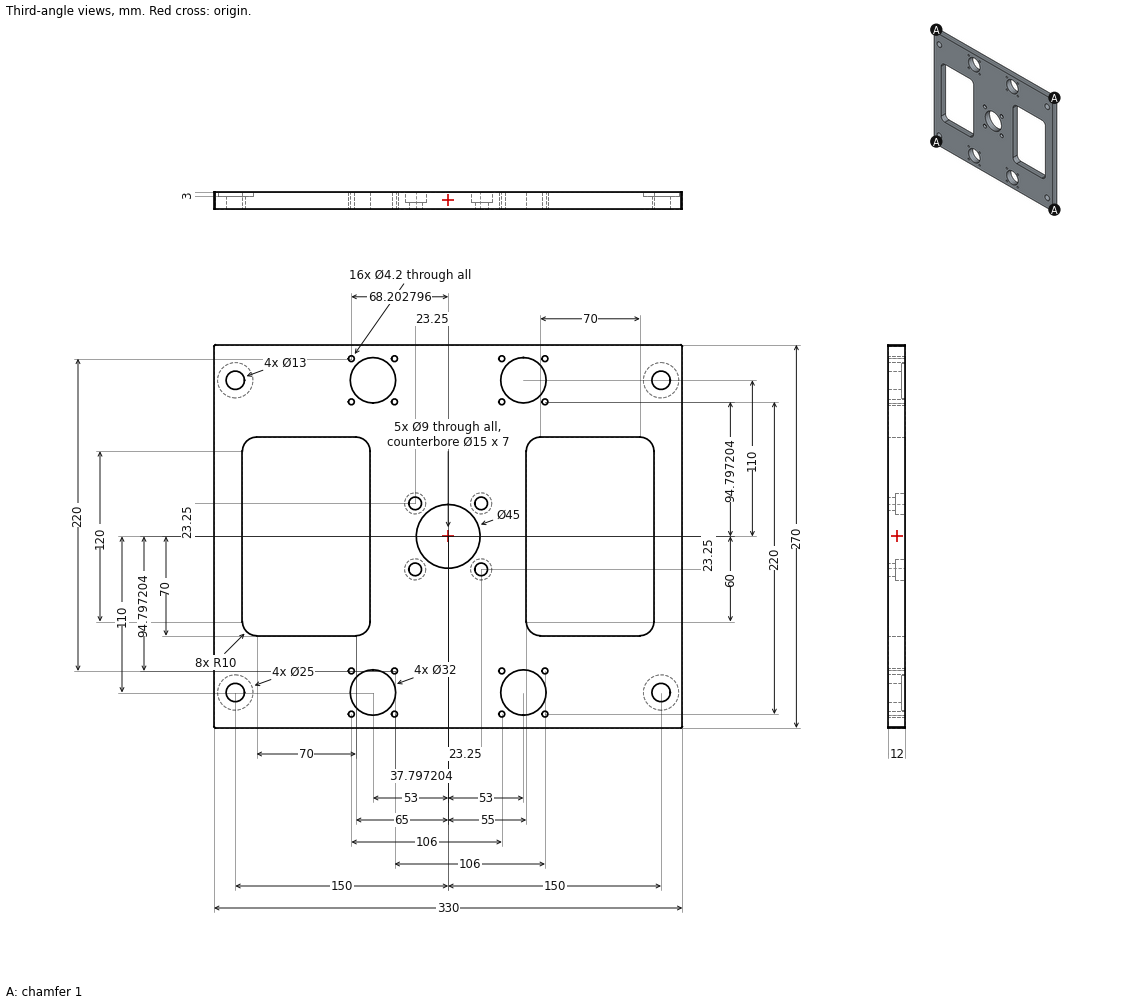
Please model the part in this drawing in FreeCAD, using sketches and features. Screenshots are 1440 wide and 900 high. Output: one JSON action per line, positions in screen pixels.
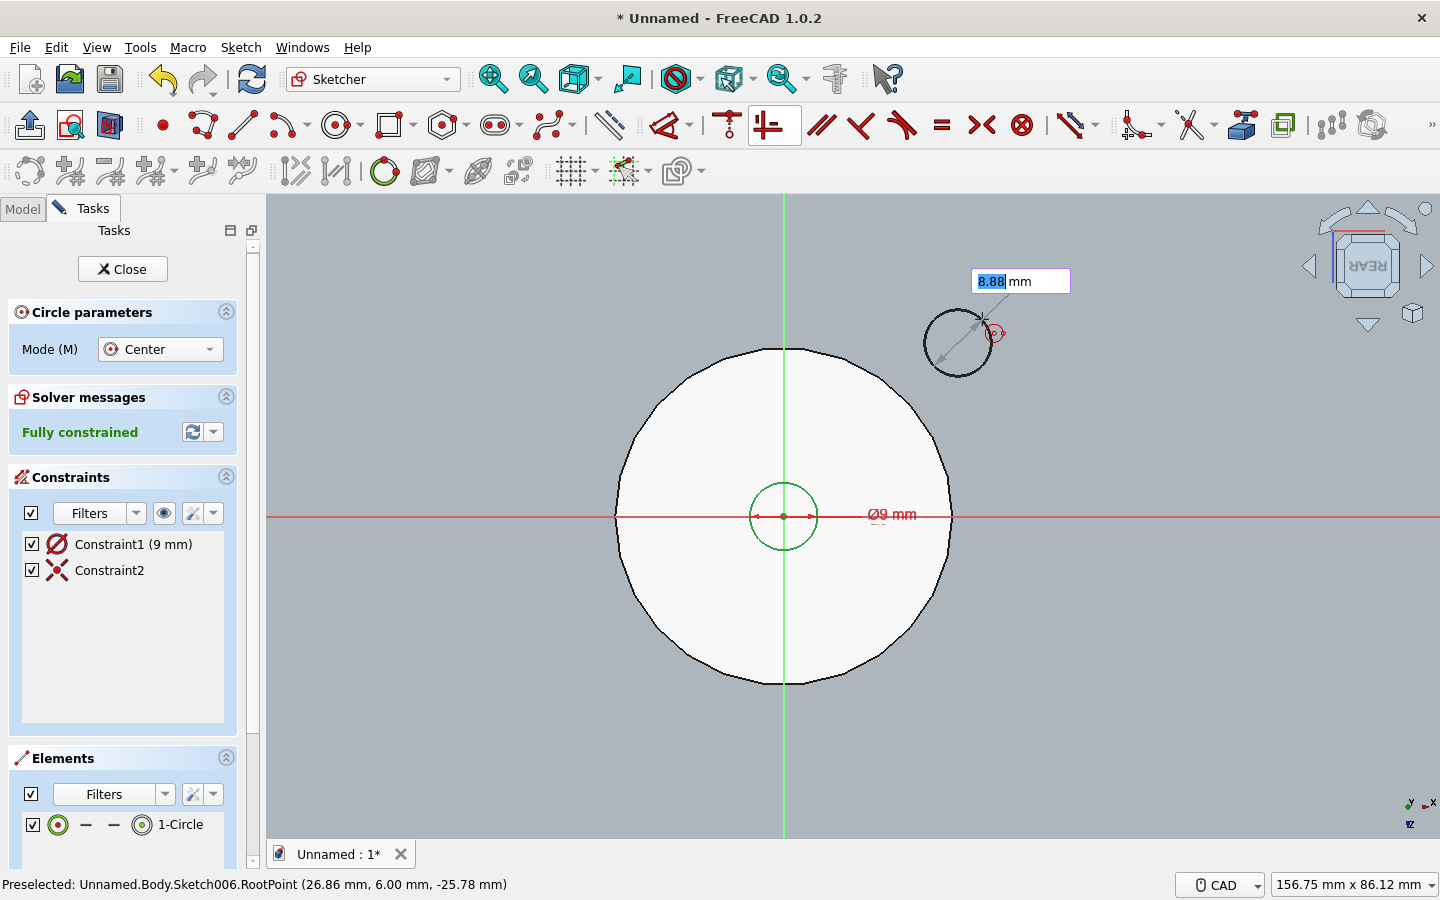
{"action": "type", "text": "9"}
{"action": "key", "text": "Return"}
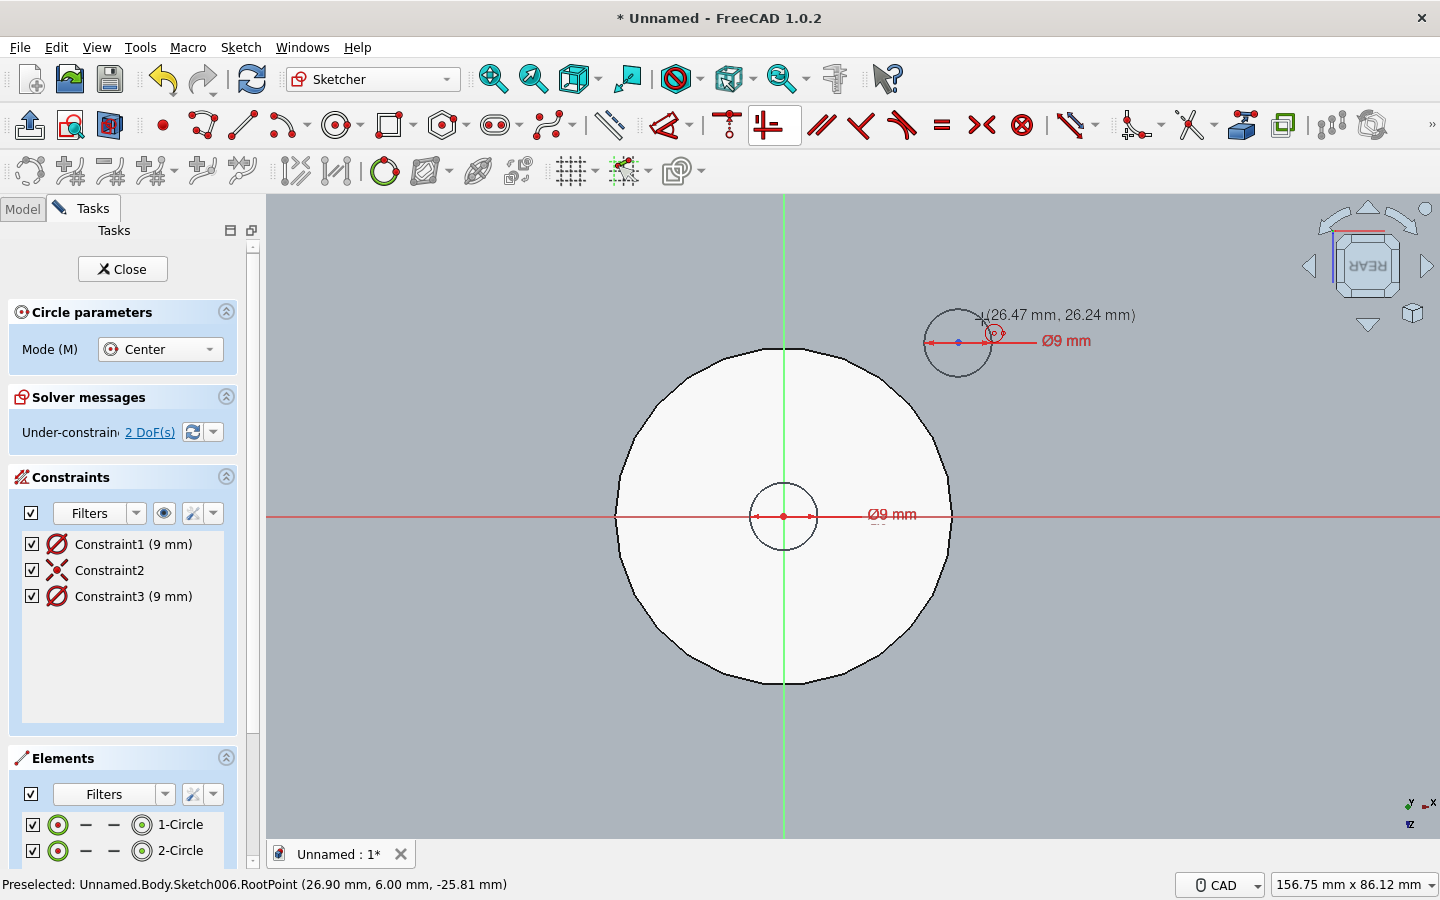
{"action": "left_click", "coordinate": [610, 691]}
{"action": "mouse_move", "coordinate": [633, 667]}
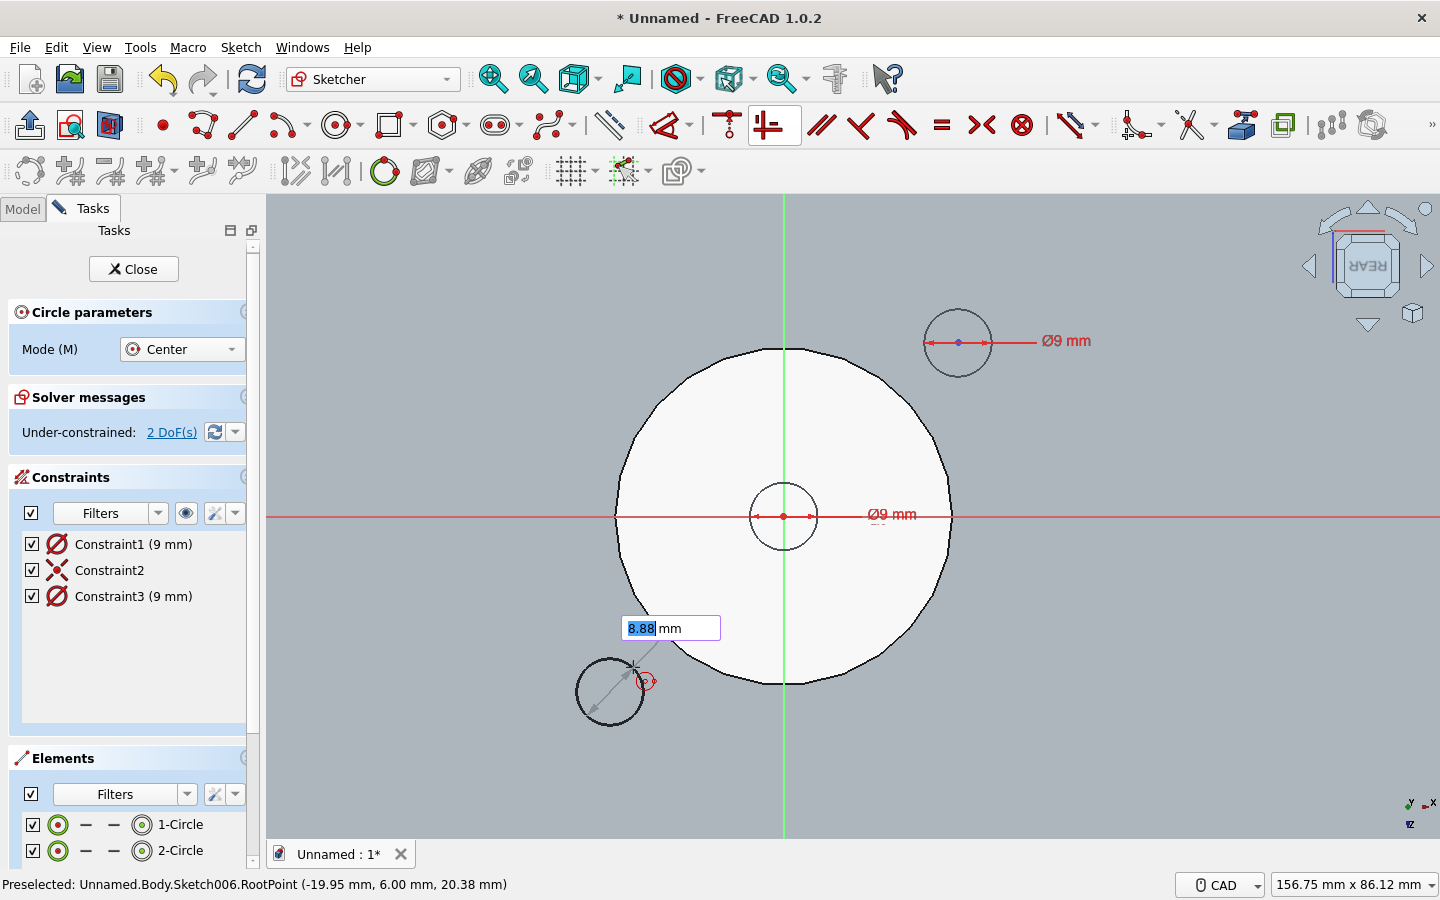
{"action": "type", "text": "9"}
{"action": "key", "text": "Return"}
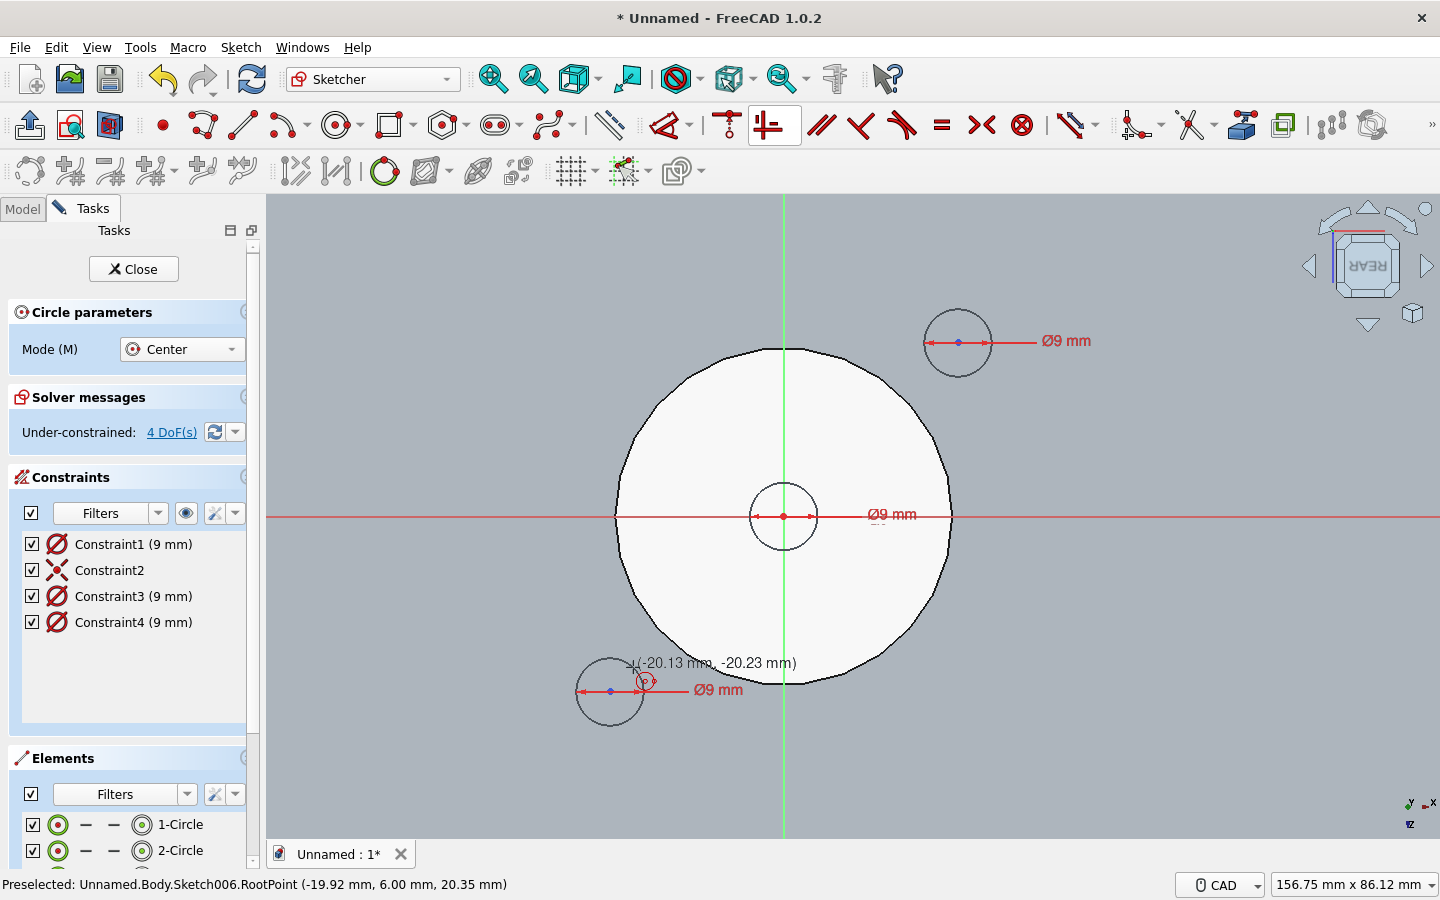
{"action": "left_click", "coordinate": [610, 342]}
{"action": "mouse_move", "coordinate": [633, 319]}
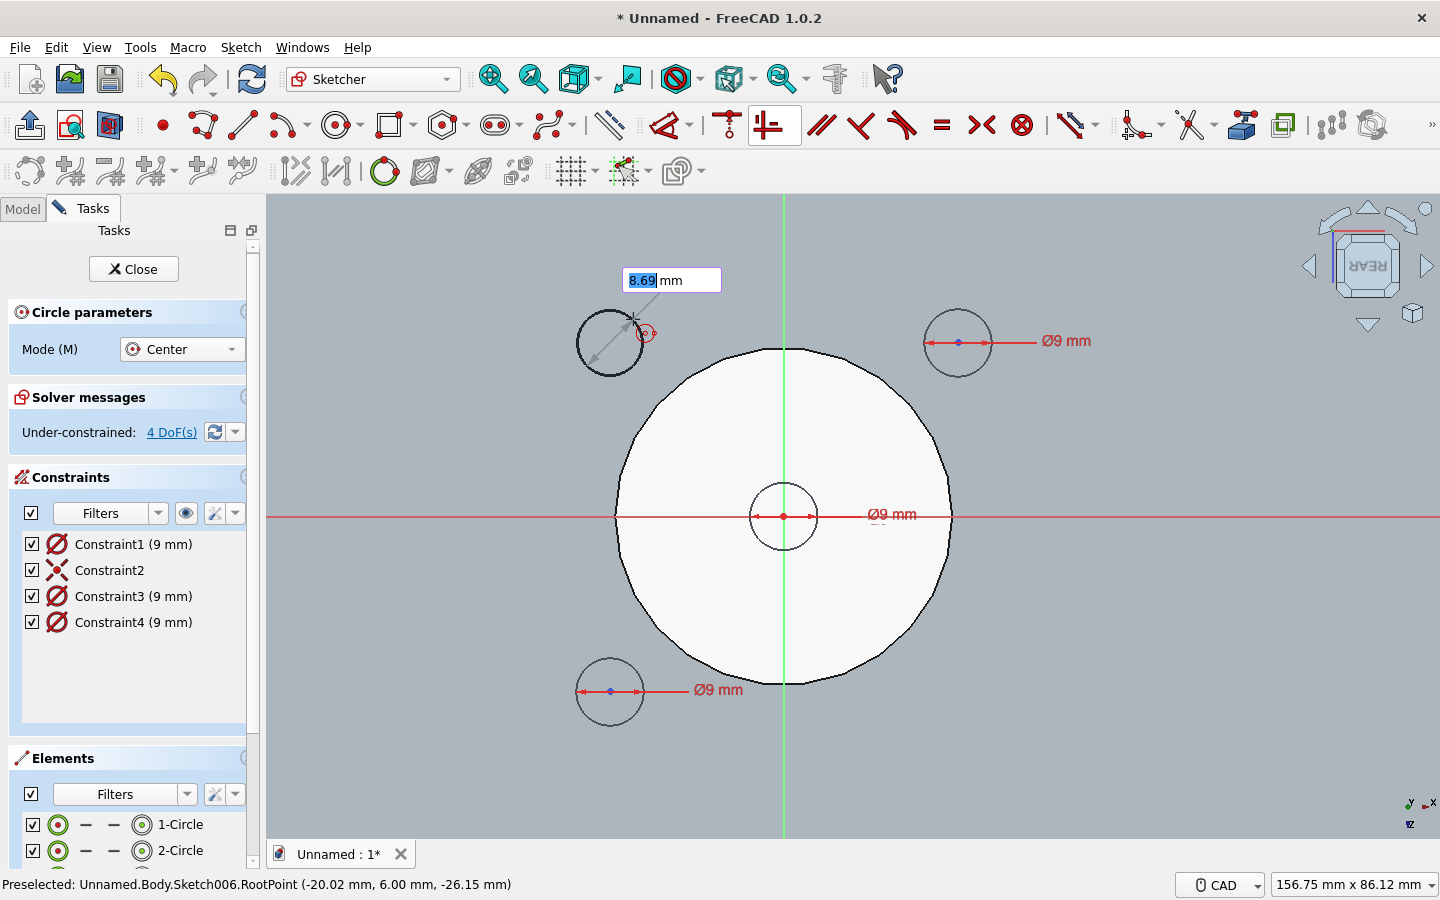
{"action": "type", "text": "9"}
{"action": "key", "text": "Return"}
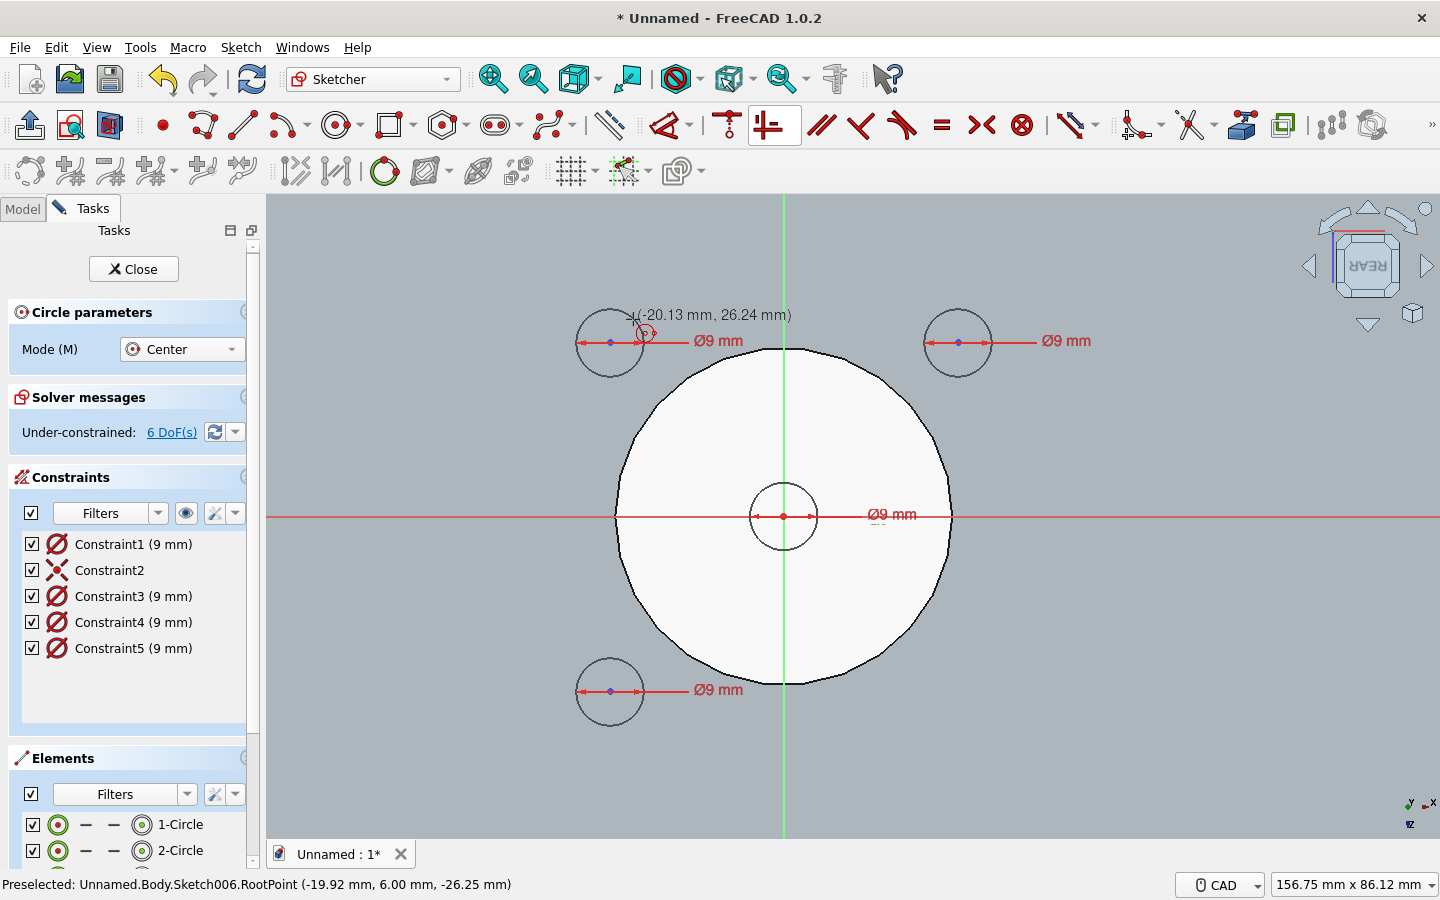
{"action": "left_click", "coordinate": [958, 691]}
{"action": "mouse_move", "coordinate": [982, 667]}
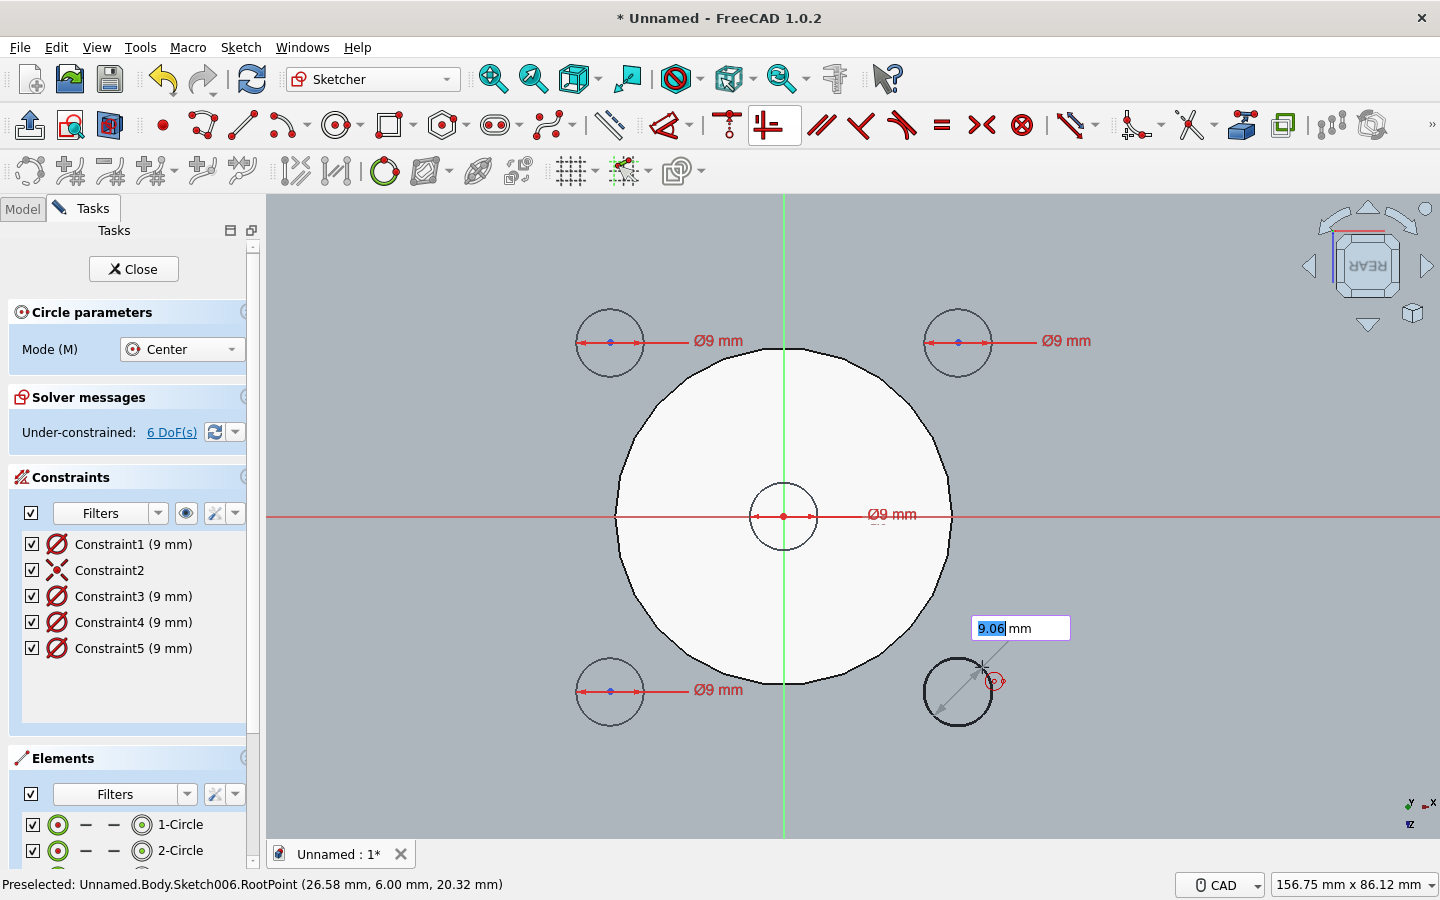
{"action": "type", "text": "9"}
{"action": "key", "text": "Return"}
{"action": "key", "text": "Escape"}